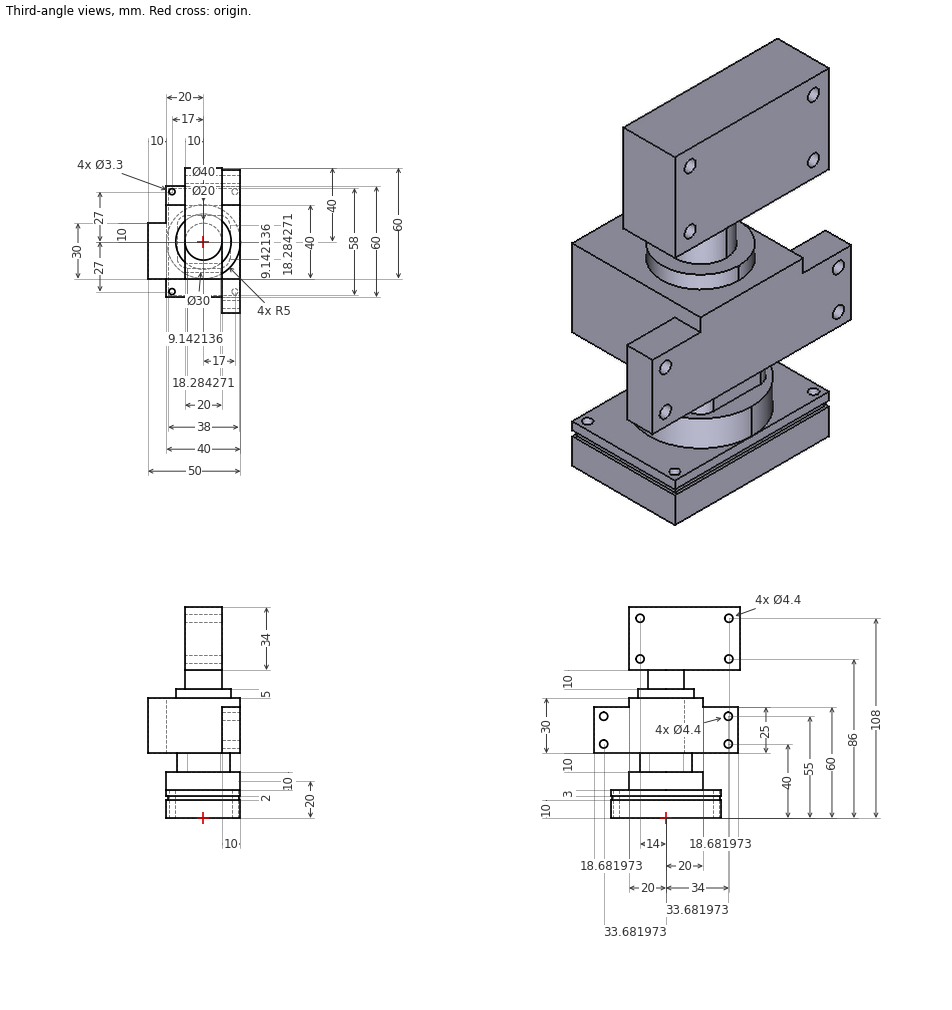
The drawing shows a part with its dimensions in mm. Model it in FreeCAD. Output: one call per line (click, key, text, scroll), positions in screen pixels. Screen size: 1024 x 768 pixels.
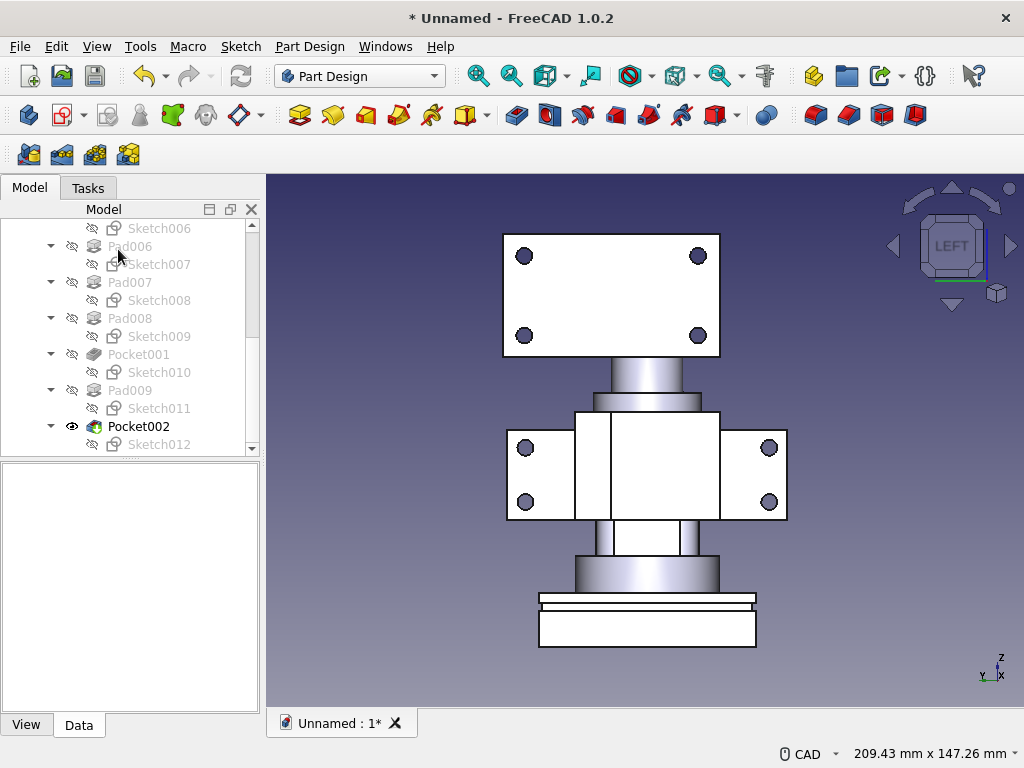
key(0)